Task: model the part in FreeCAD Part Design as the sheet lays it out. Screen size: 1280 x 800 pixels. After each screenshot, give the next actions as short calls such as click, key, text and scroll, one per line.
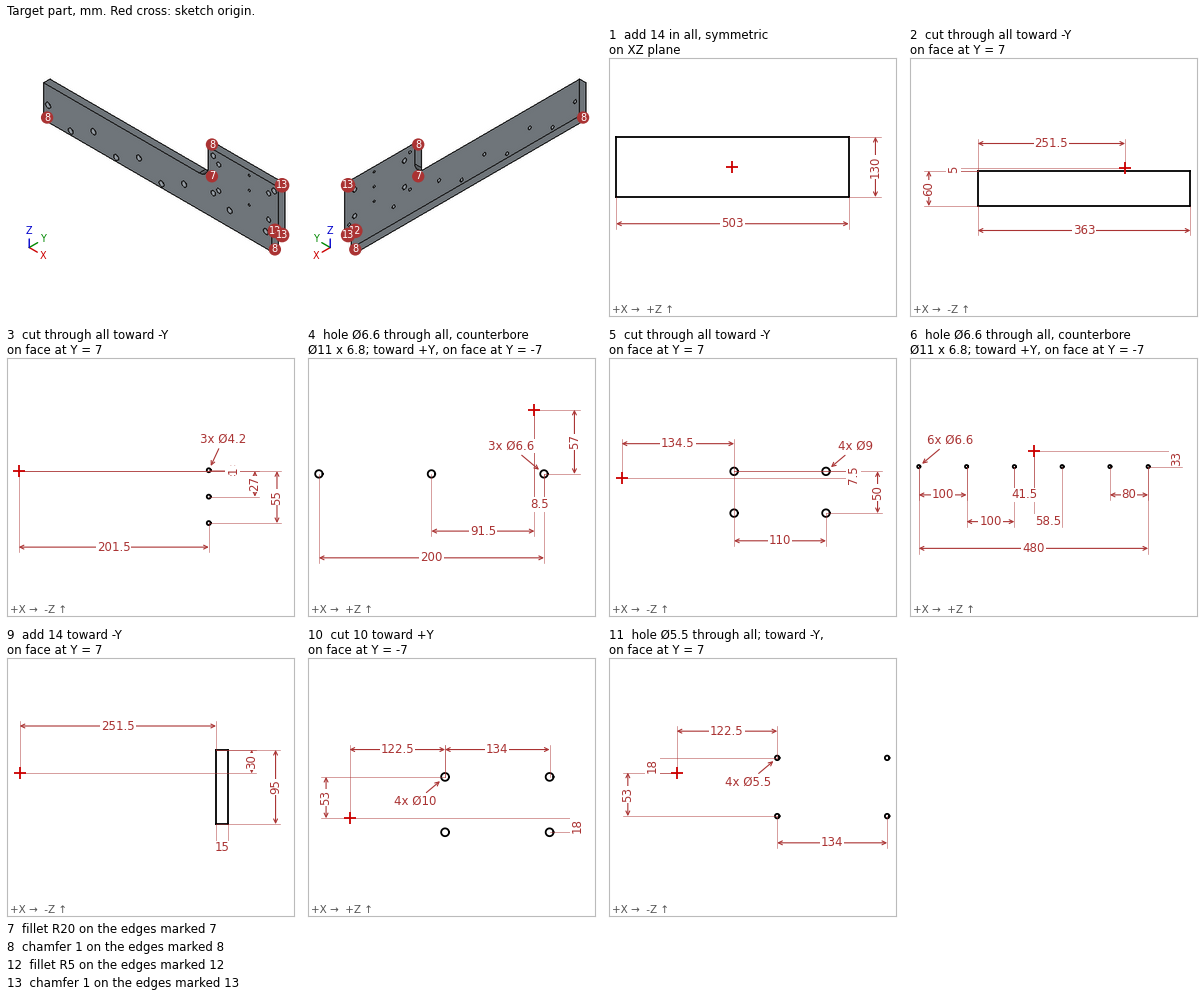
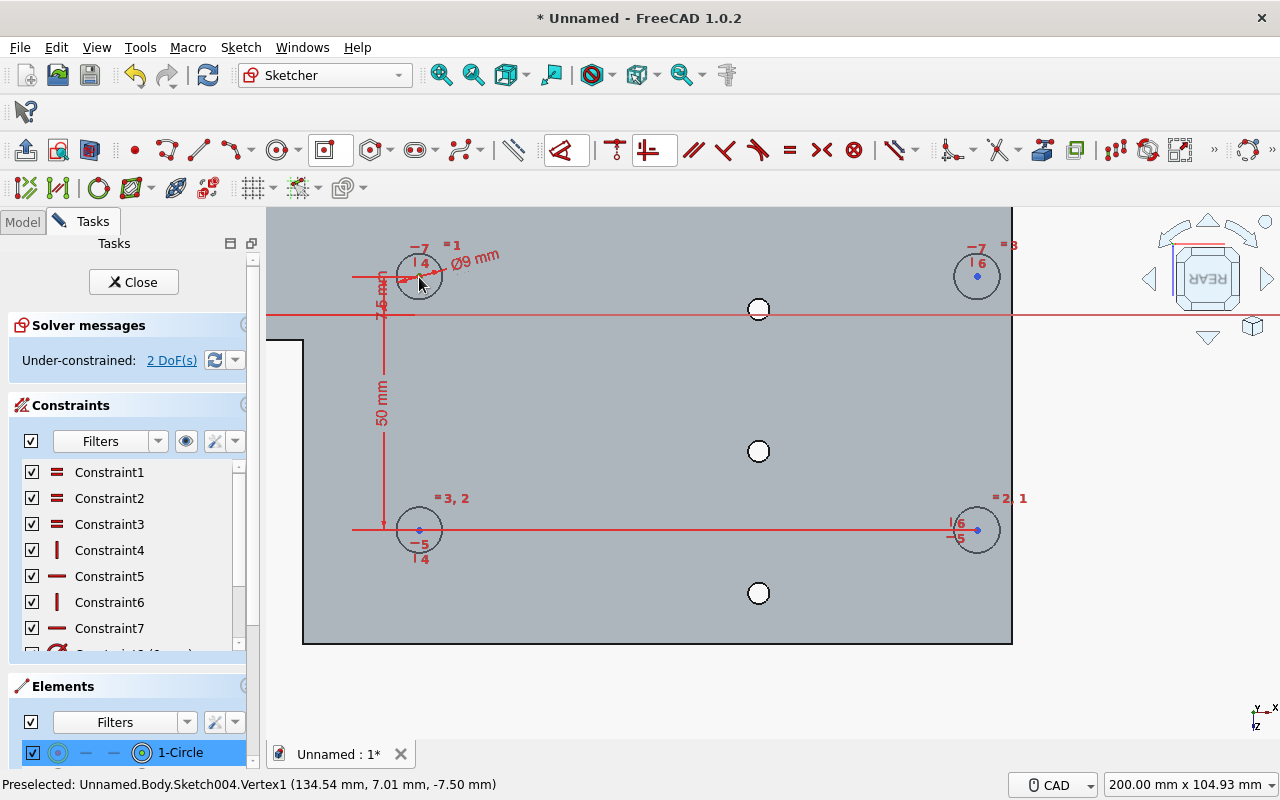
click(977, 530)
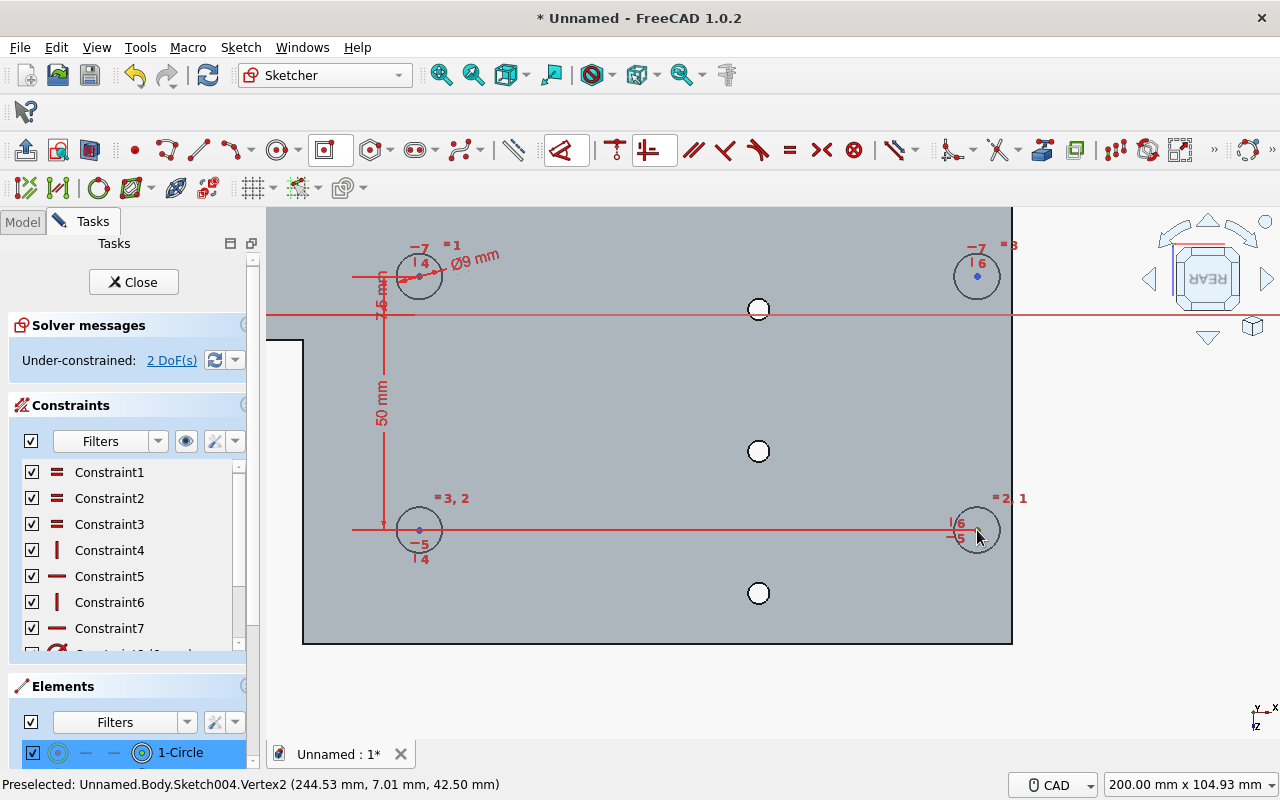
key(l)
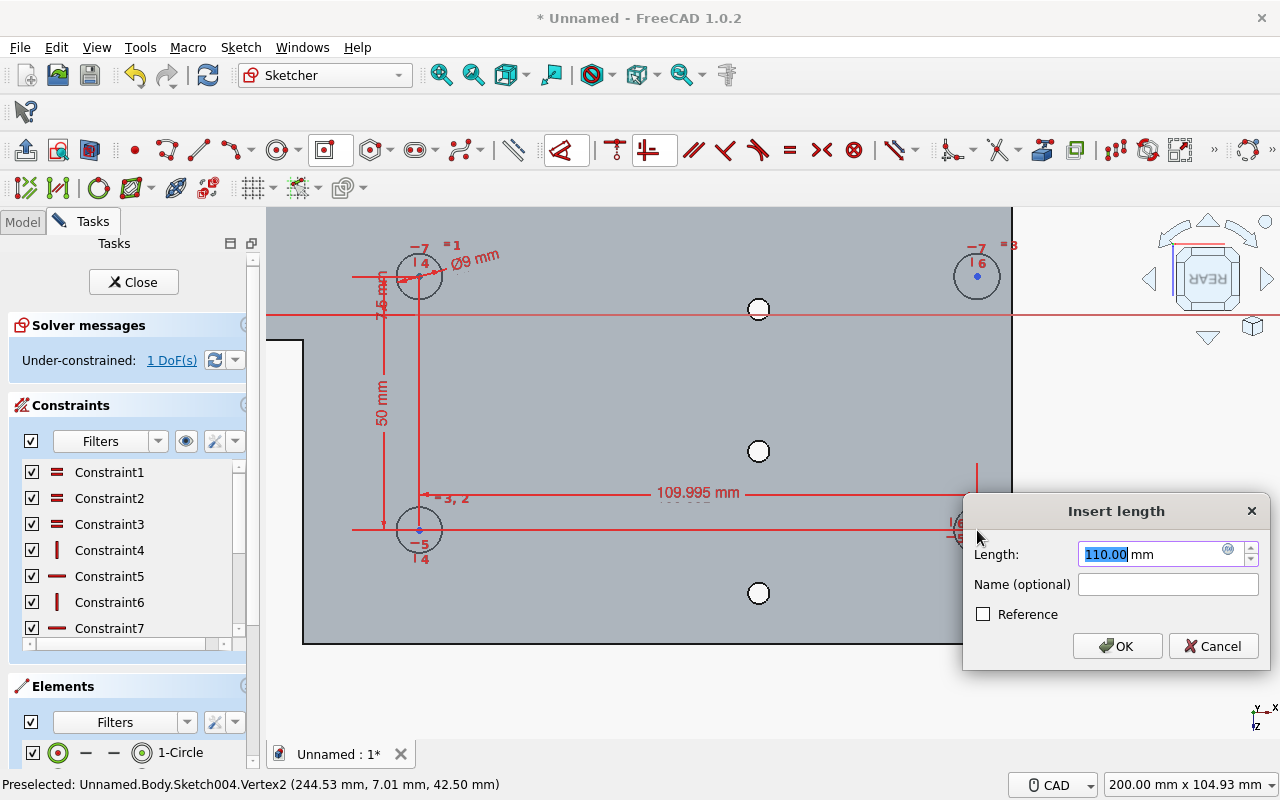
text(110)
key(Return)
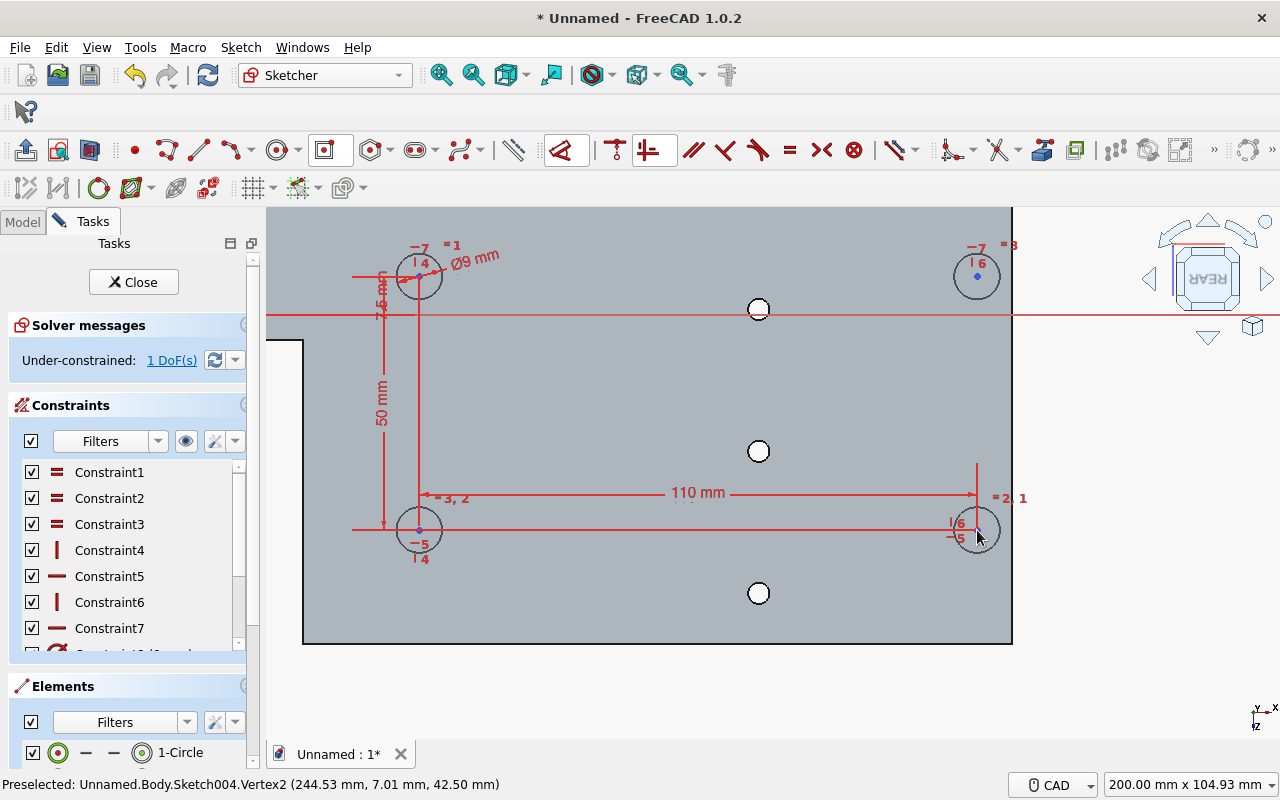
click(419, 277)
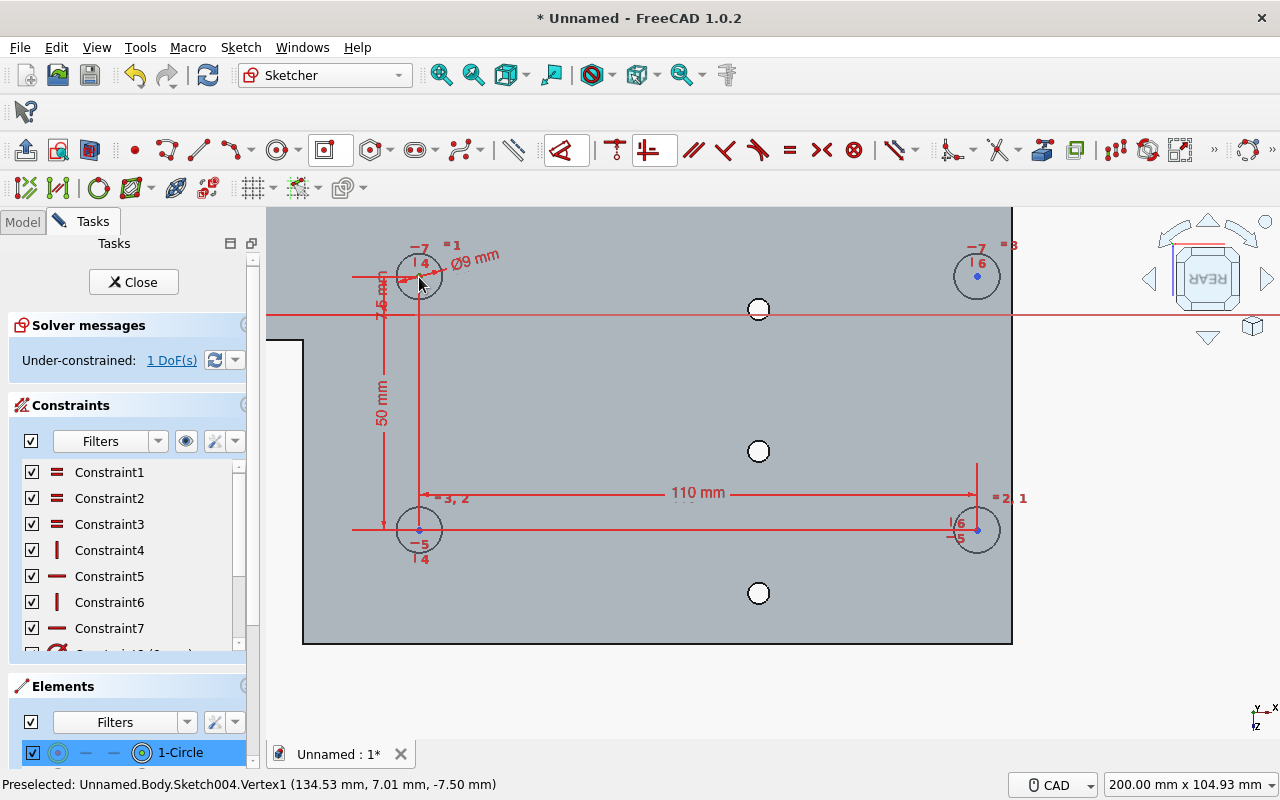
click(584, 150)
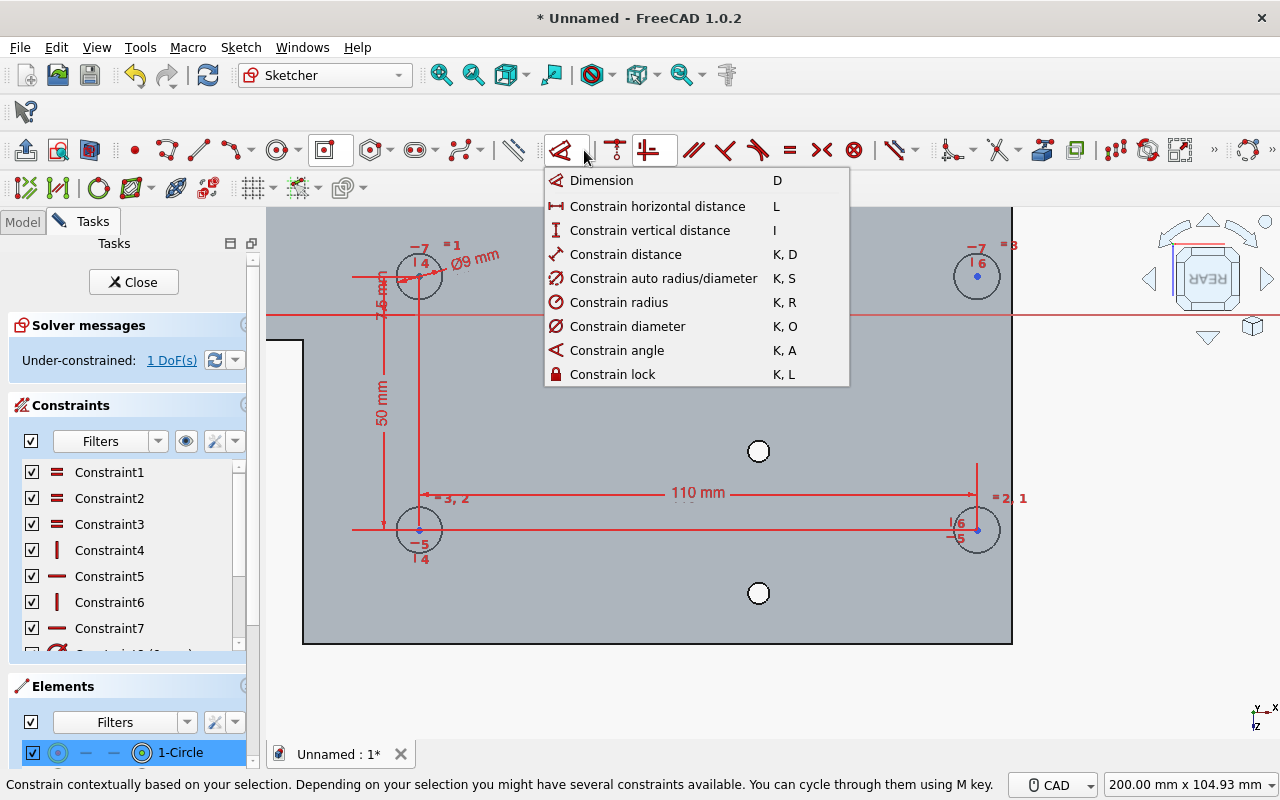
click(697, 206)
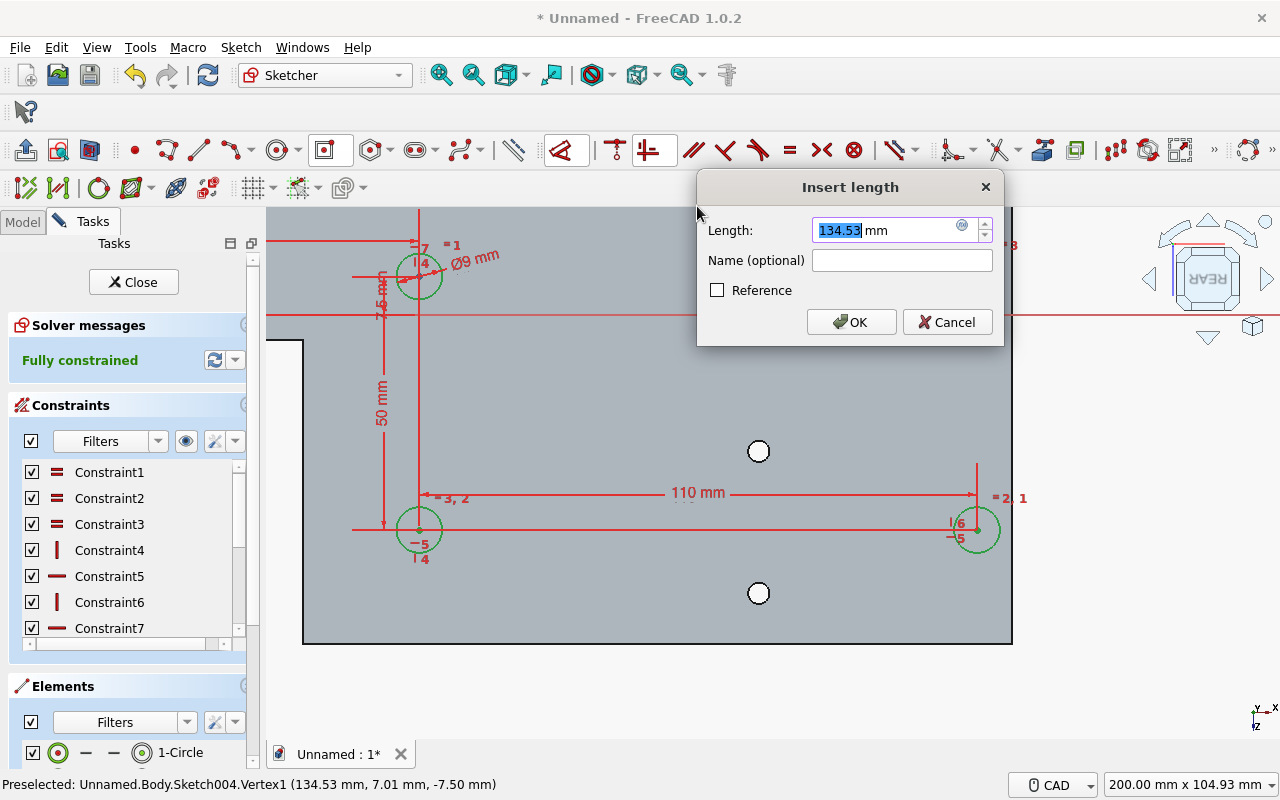
text(134.5)
key(Return)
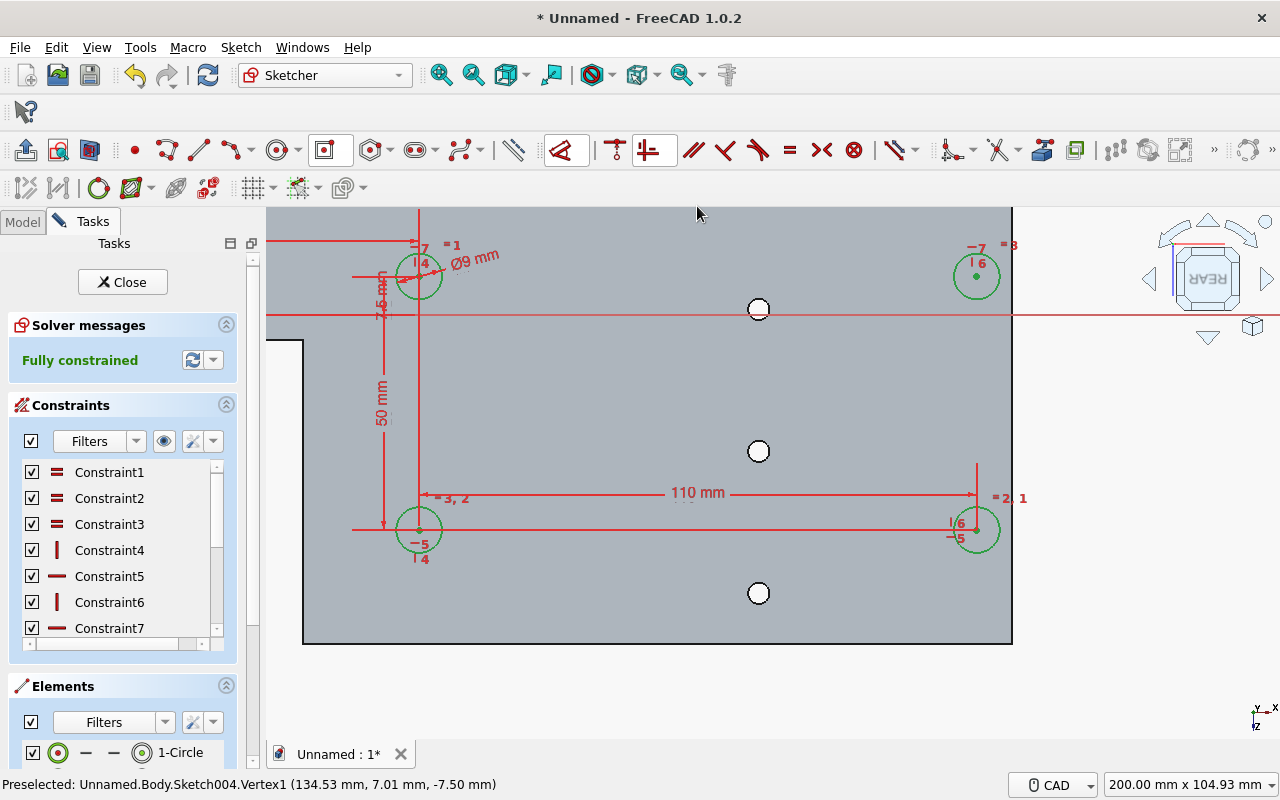
click(123, 282)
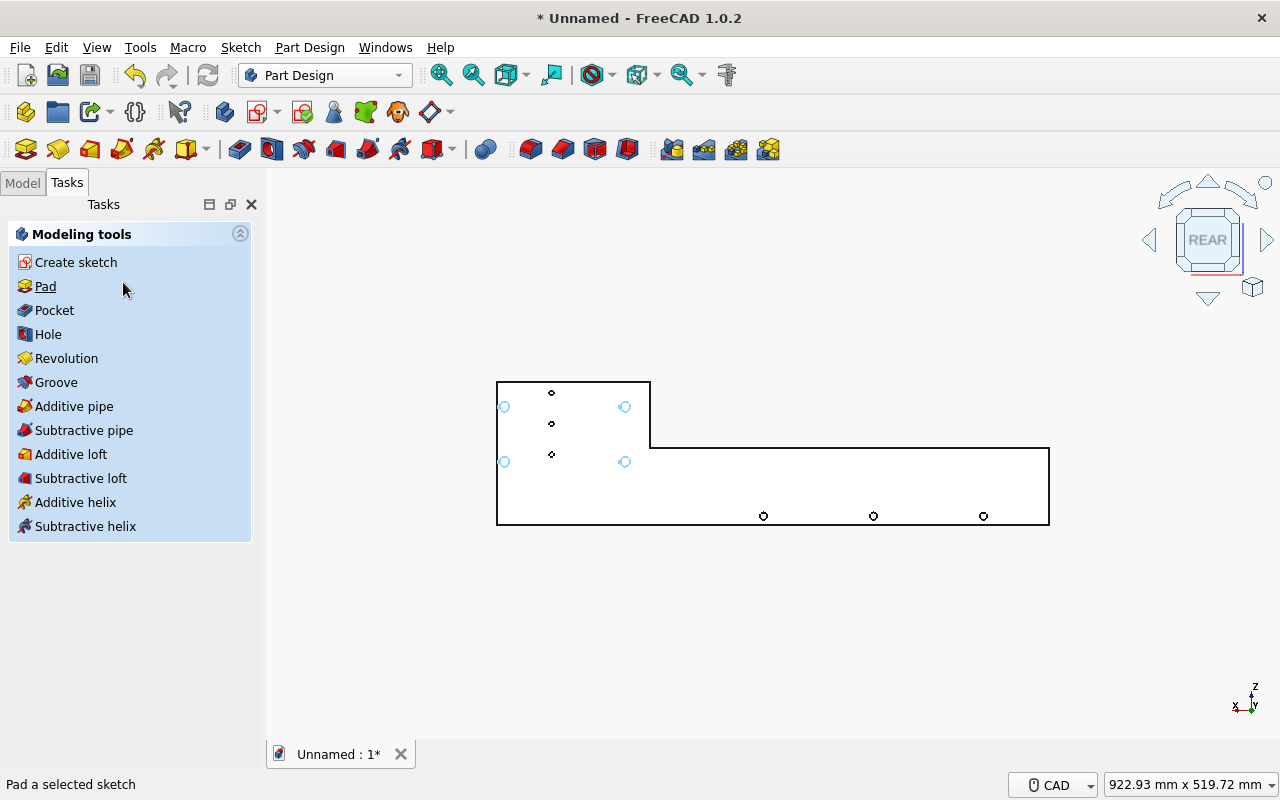
click(240, 150)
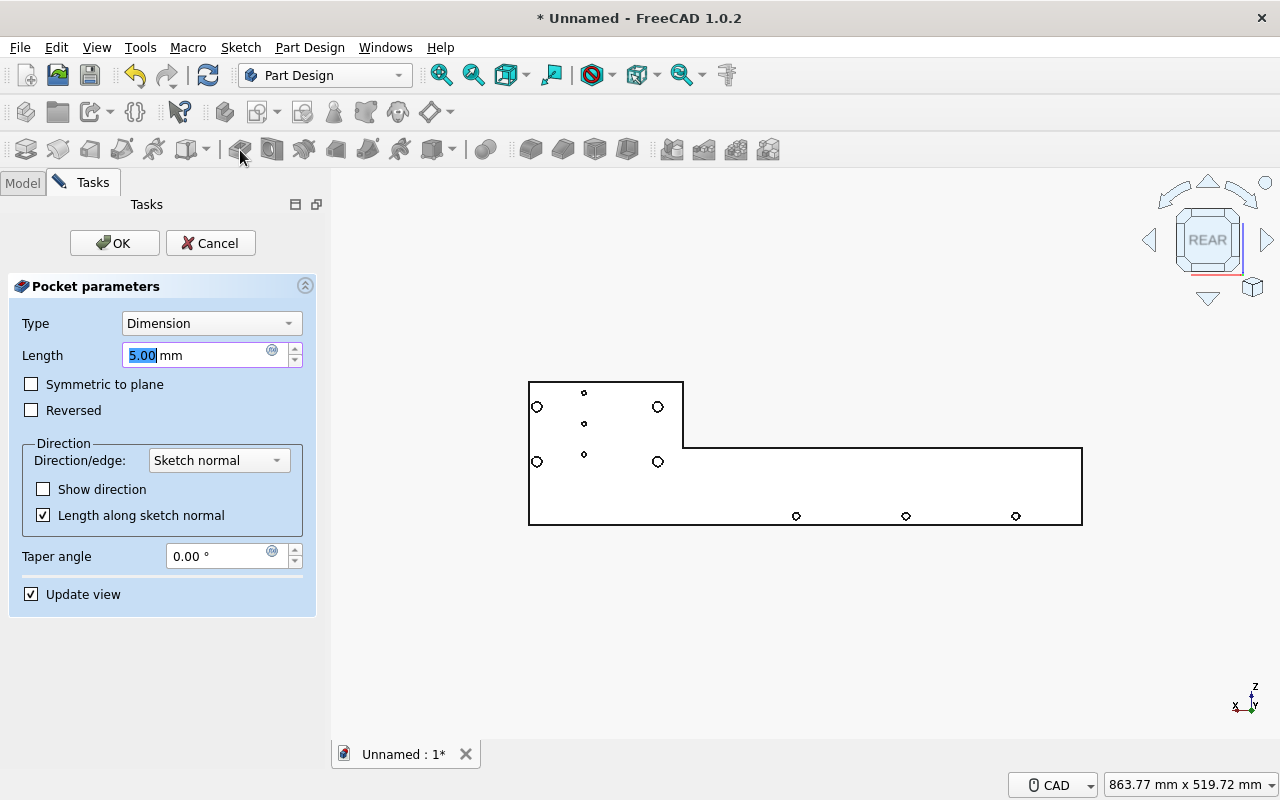
click(212, 324)